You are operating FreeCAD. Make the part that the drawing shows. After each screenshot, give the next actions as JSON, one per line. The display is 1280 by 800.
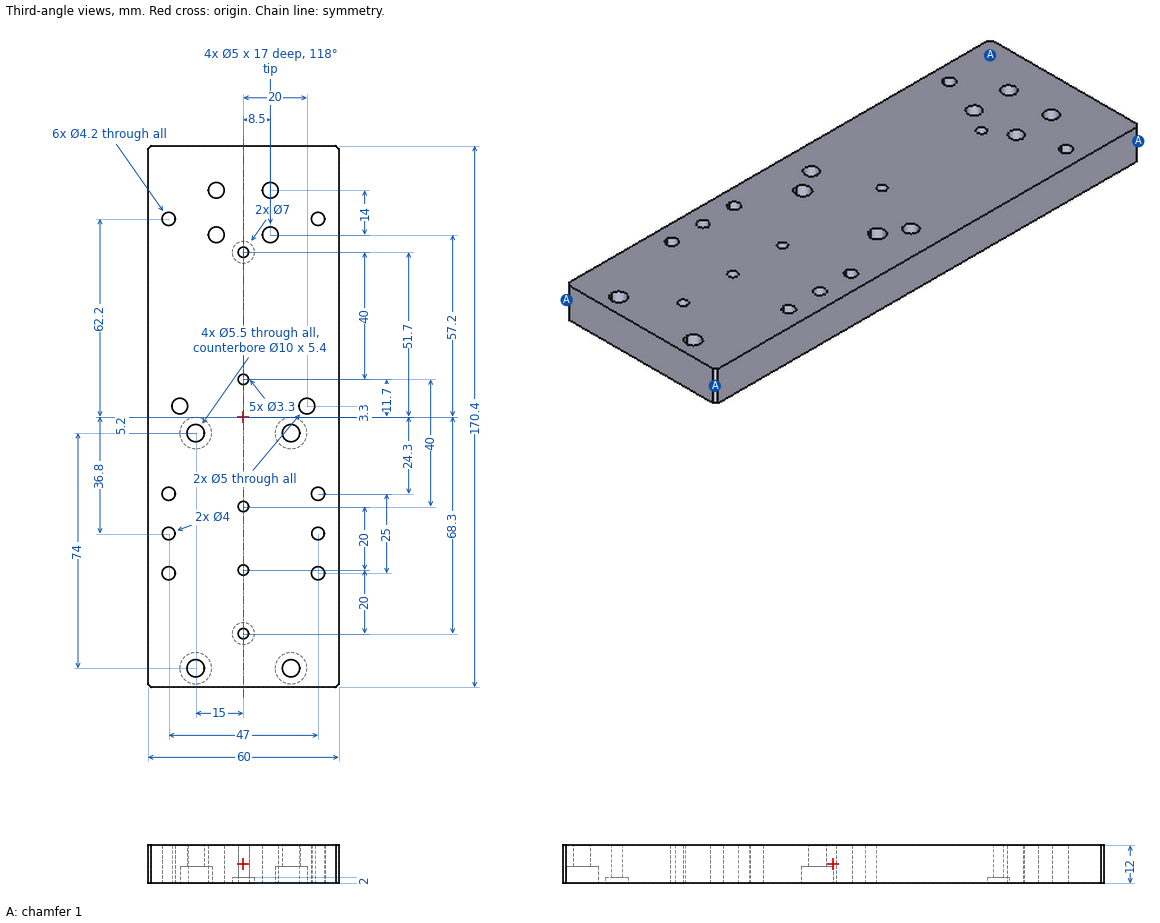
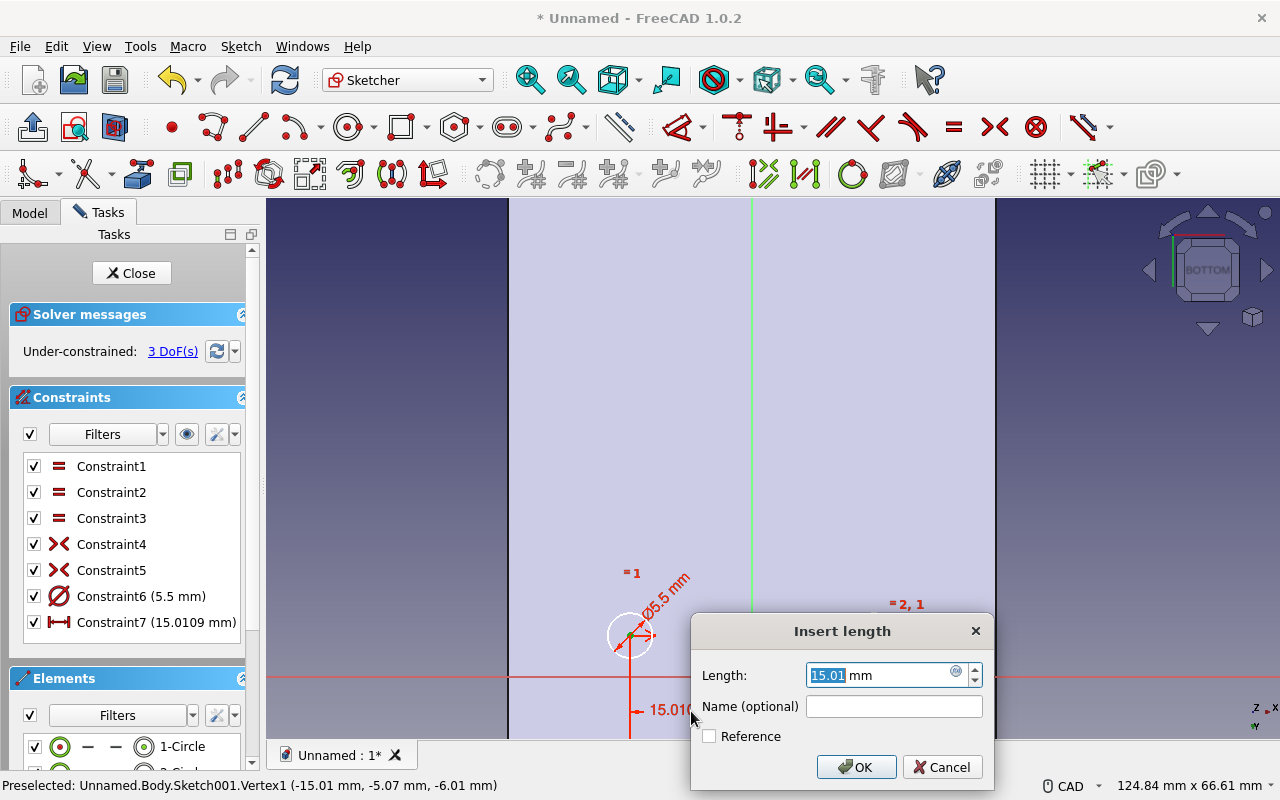
{"action": "type", "text": "15"}
{"action": "key", "text": "Return"}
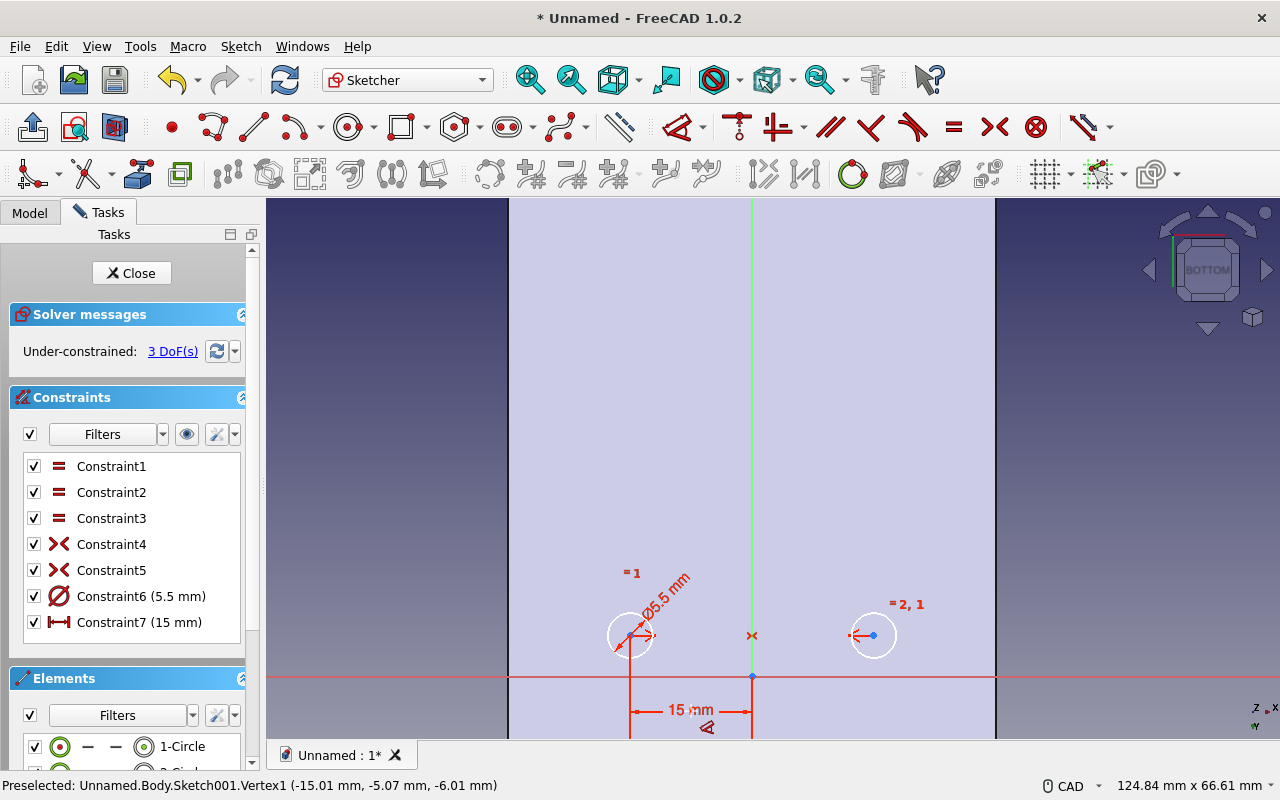
{"action": "scroll", "coordinate": [647, 620], "scroll_direction": "down", "scroll_amount": 3}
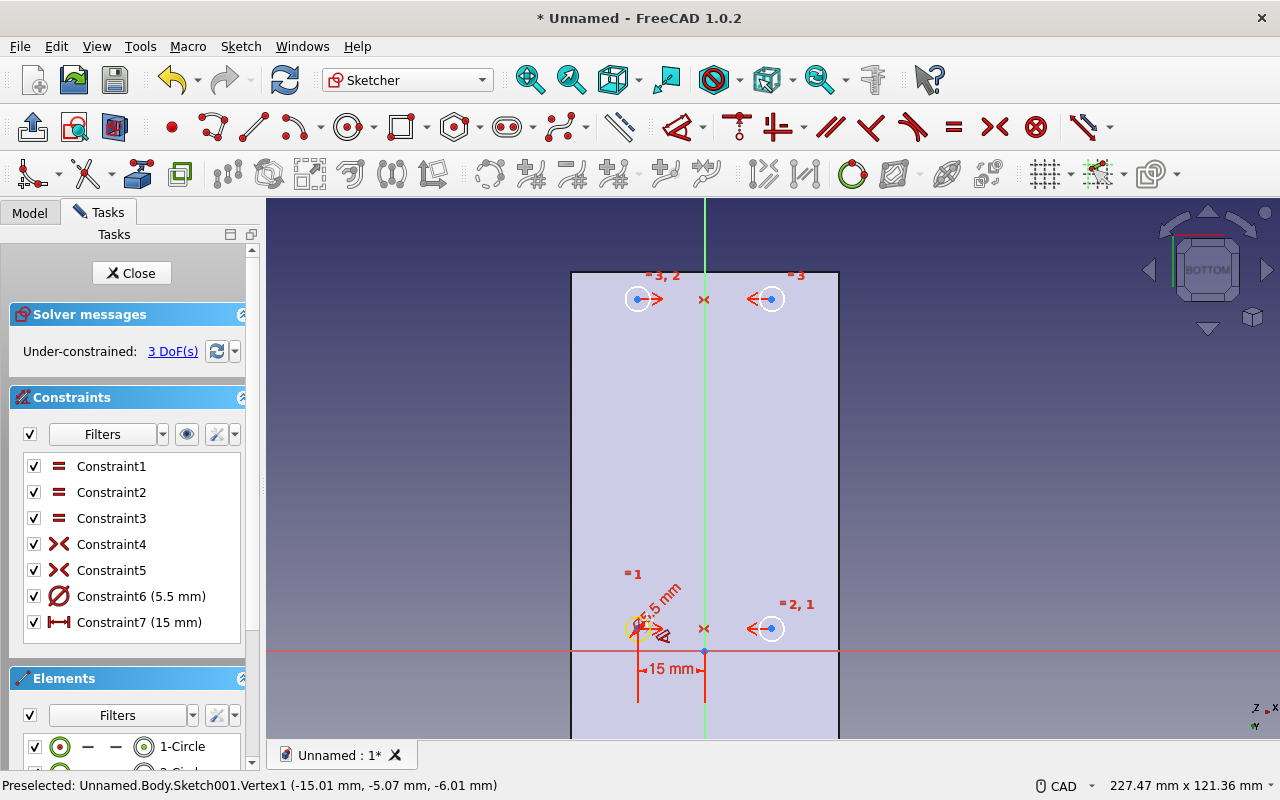
{"action": "left_click", "coordinate": [638, 299]}
{"action": "left_click", "coordinate": [671, 265]}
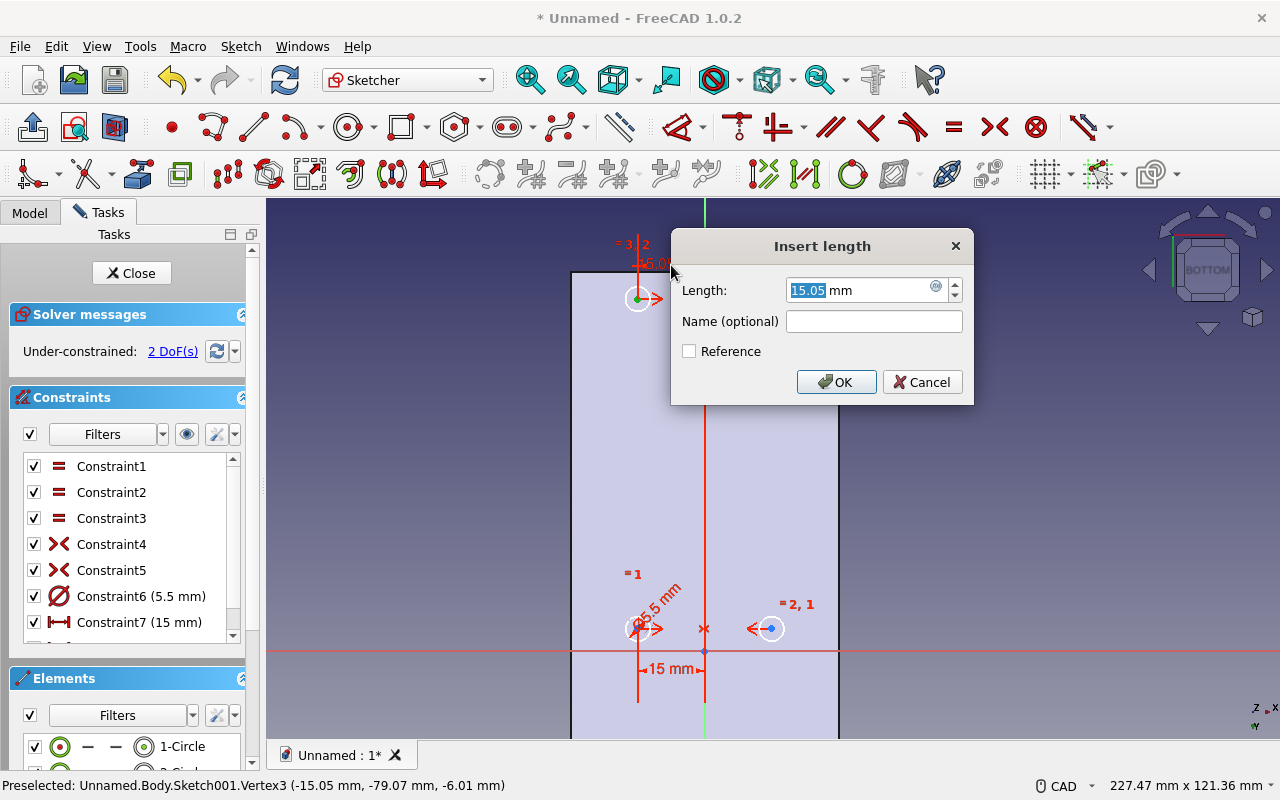
{"action": "type", "text": "15"}
{"action": "key", "text": "Return"}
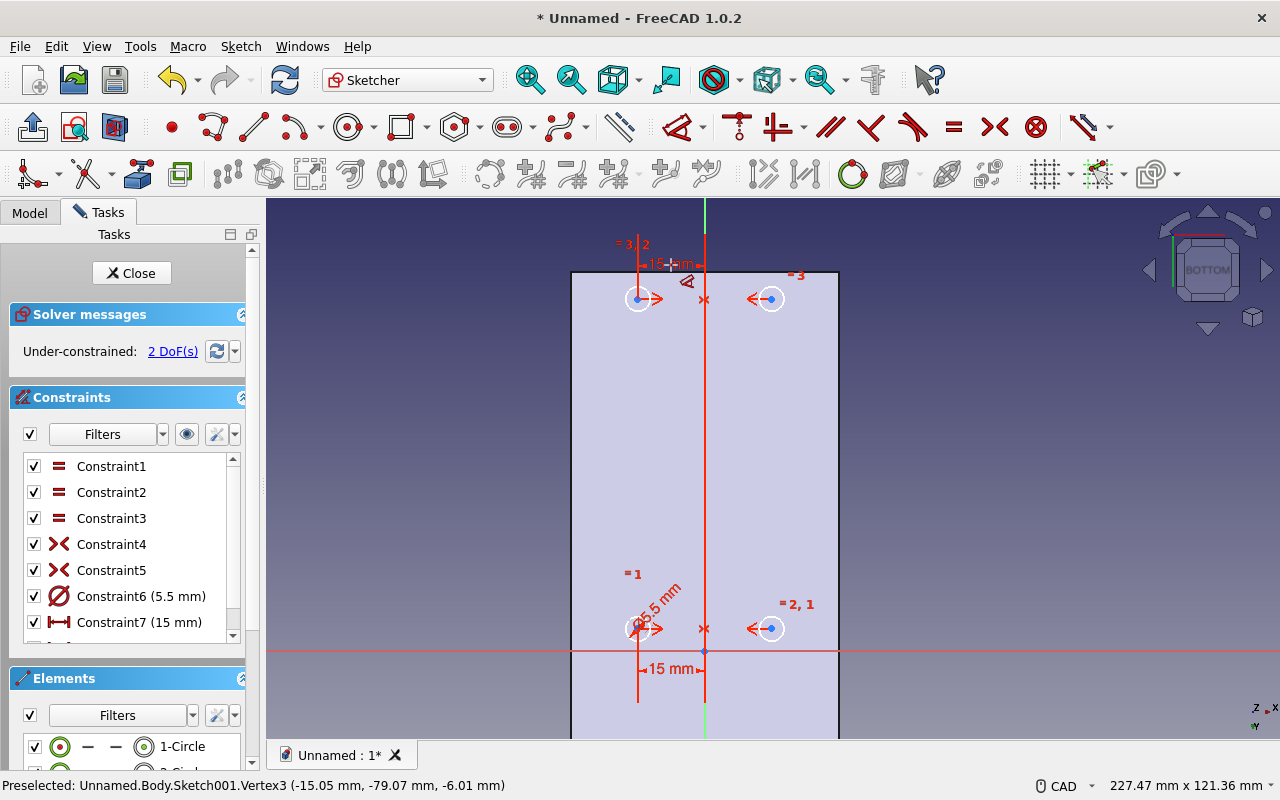
{"action": "scroll", "coordinate": [638, 629], "scroll_direction": "up", "scroll_amount": 3}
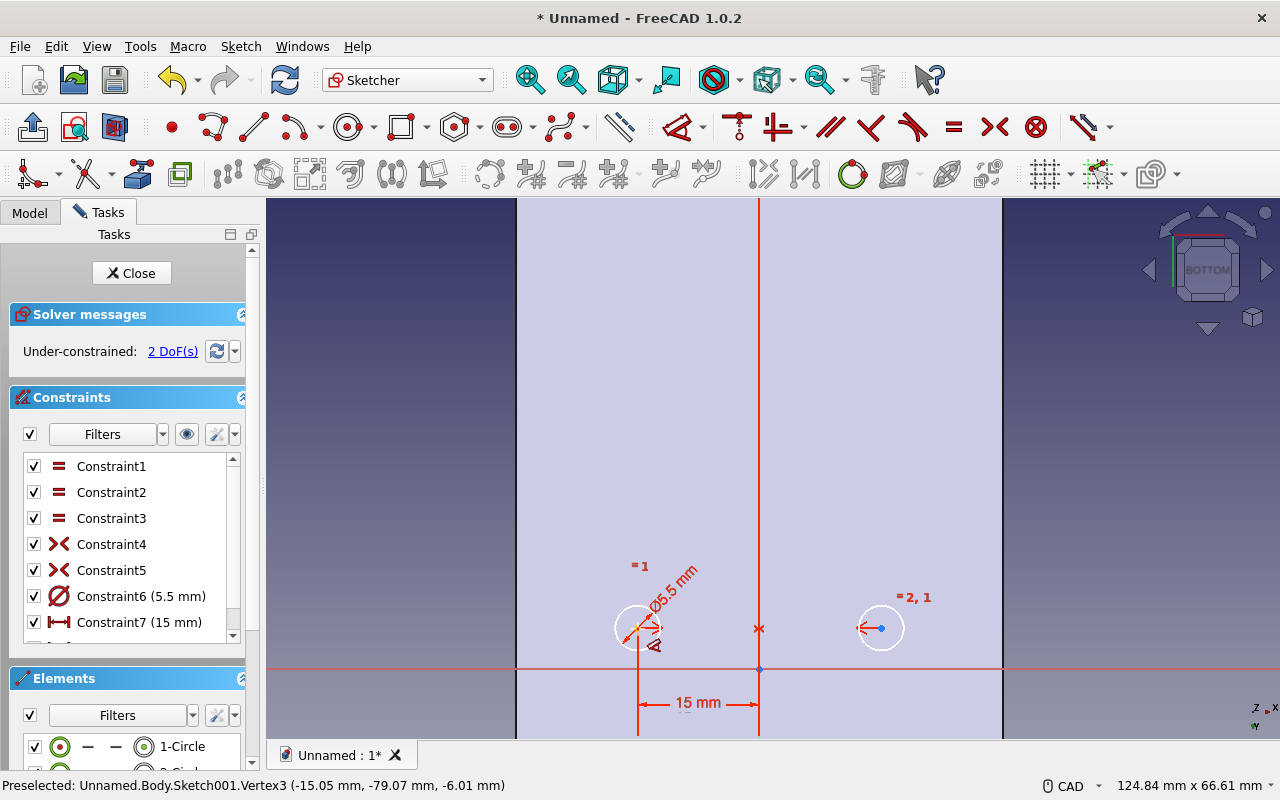
{"action": "left_click", "coordinate": [638, 628]}
{"action": "left_click", "coordinate": [604, 649]}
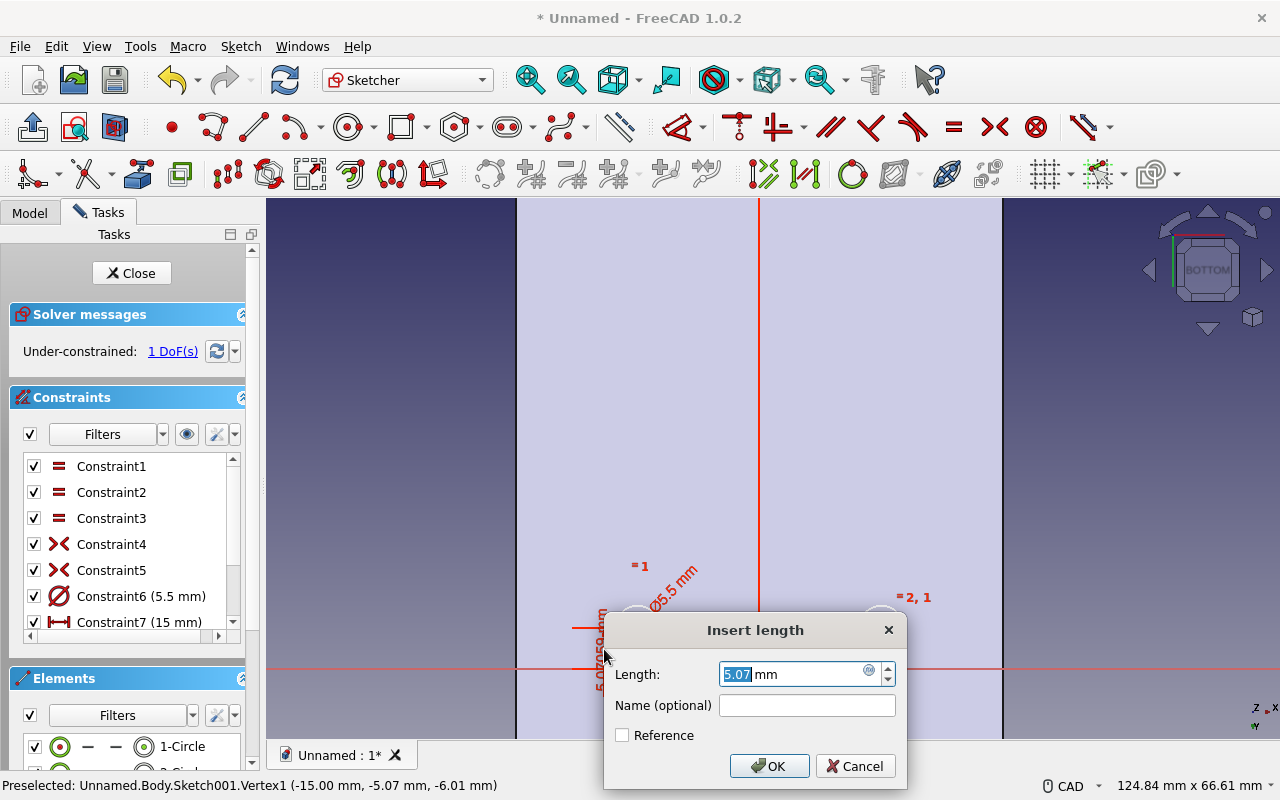
{"action": "type", "text": "5.2"}
{"action": "key", "text": "Return"}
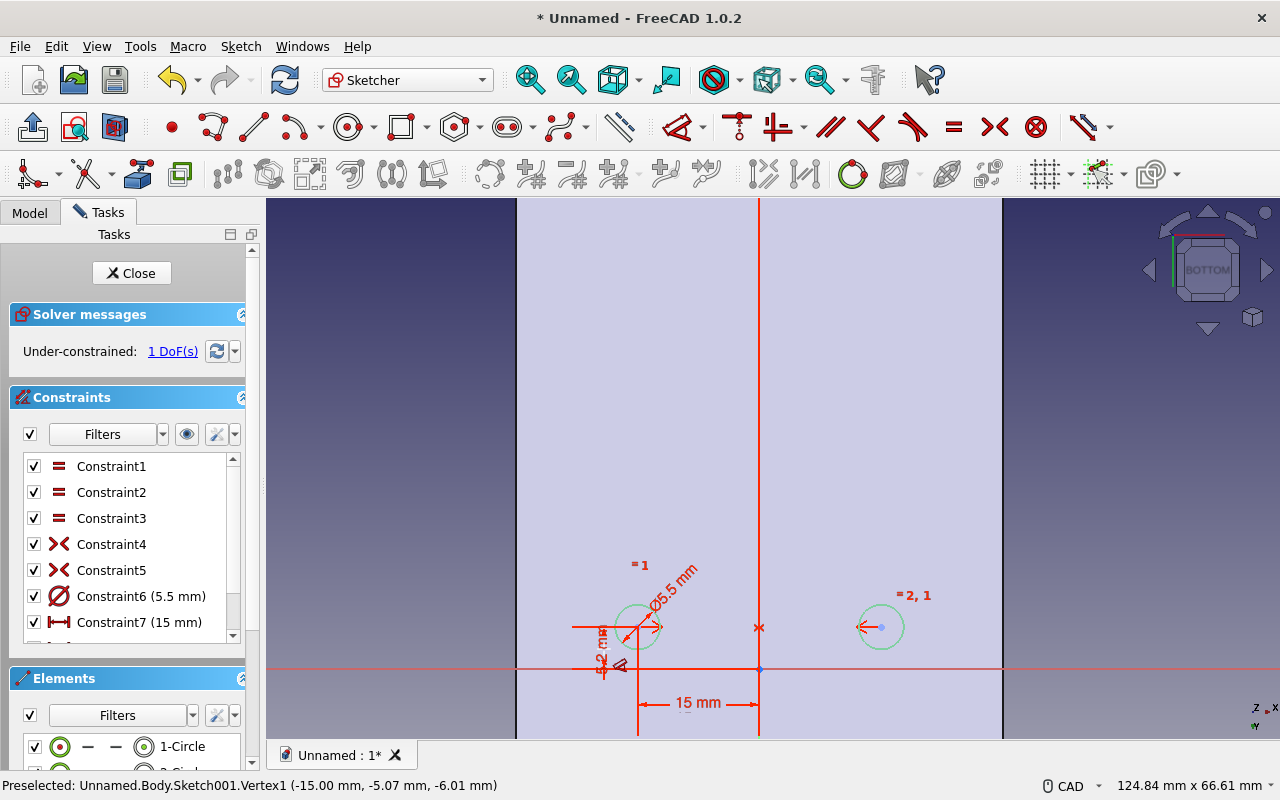
{"action": "left_click", "coordinate": [638, 627]}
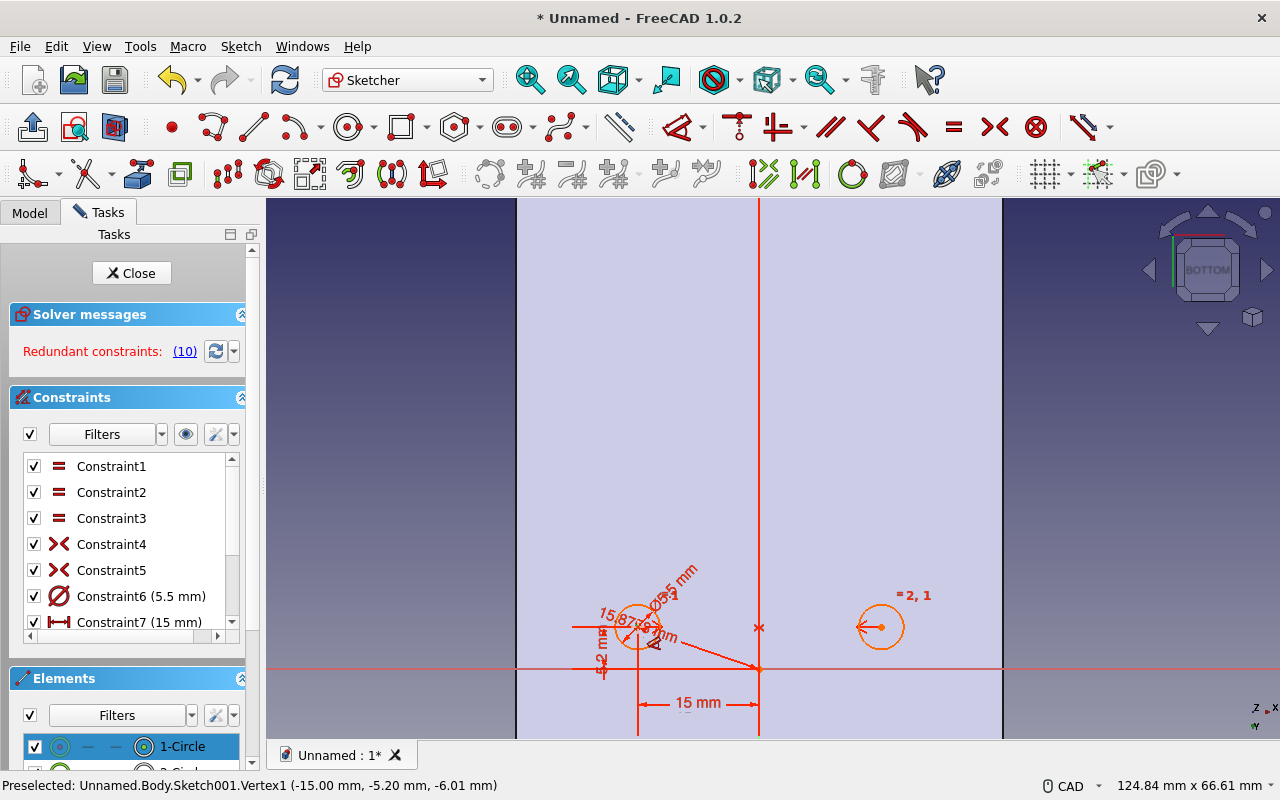
{"action": "scroll", "coordinate": [638, 629], "scroll_direction": "down", "scroll_amount": 3}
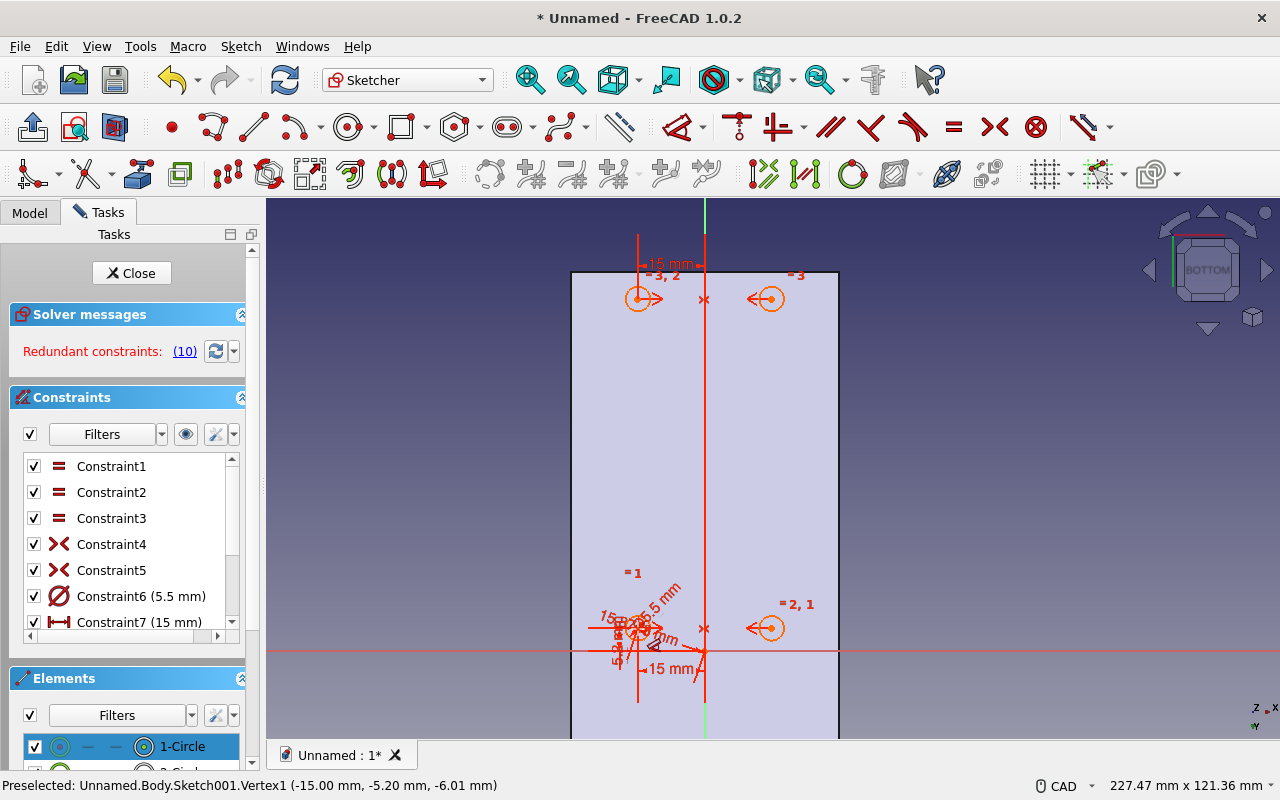
{"action": "left_click", "coordinate": [638, 299]}
{"action": "left_click", "coordinate": [604, 464]}